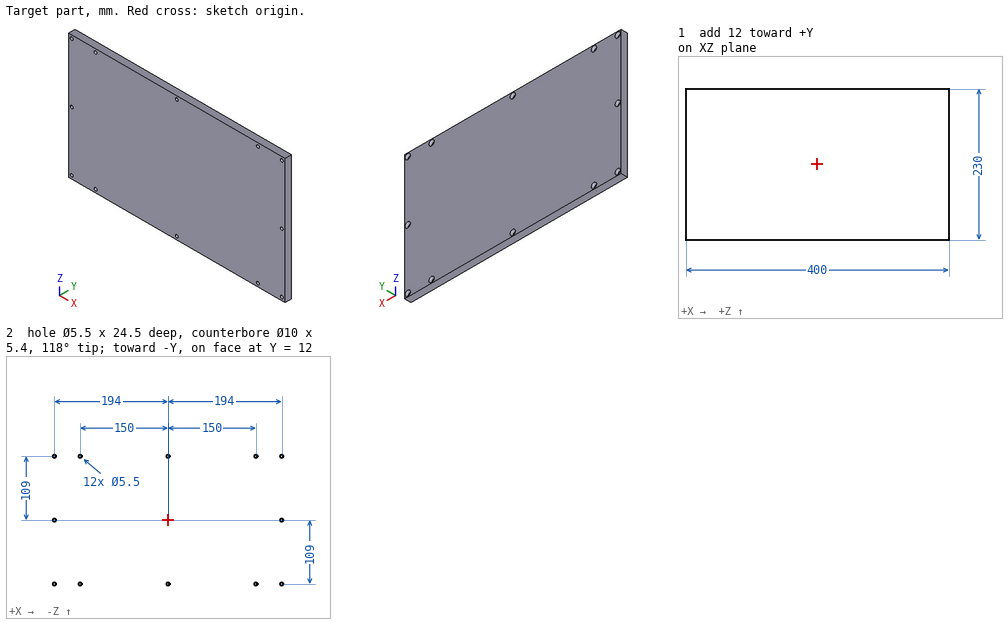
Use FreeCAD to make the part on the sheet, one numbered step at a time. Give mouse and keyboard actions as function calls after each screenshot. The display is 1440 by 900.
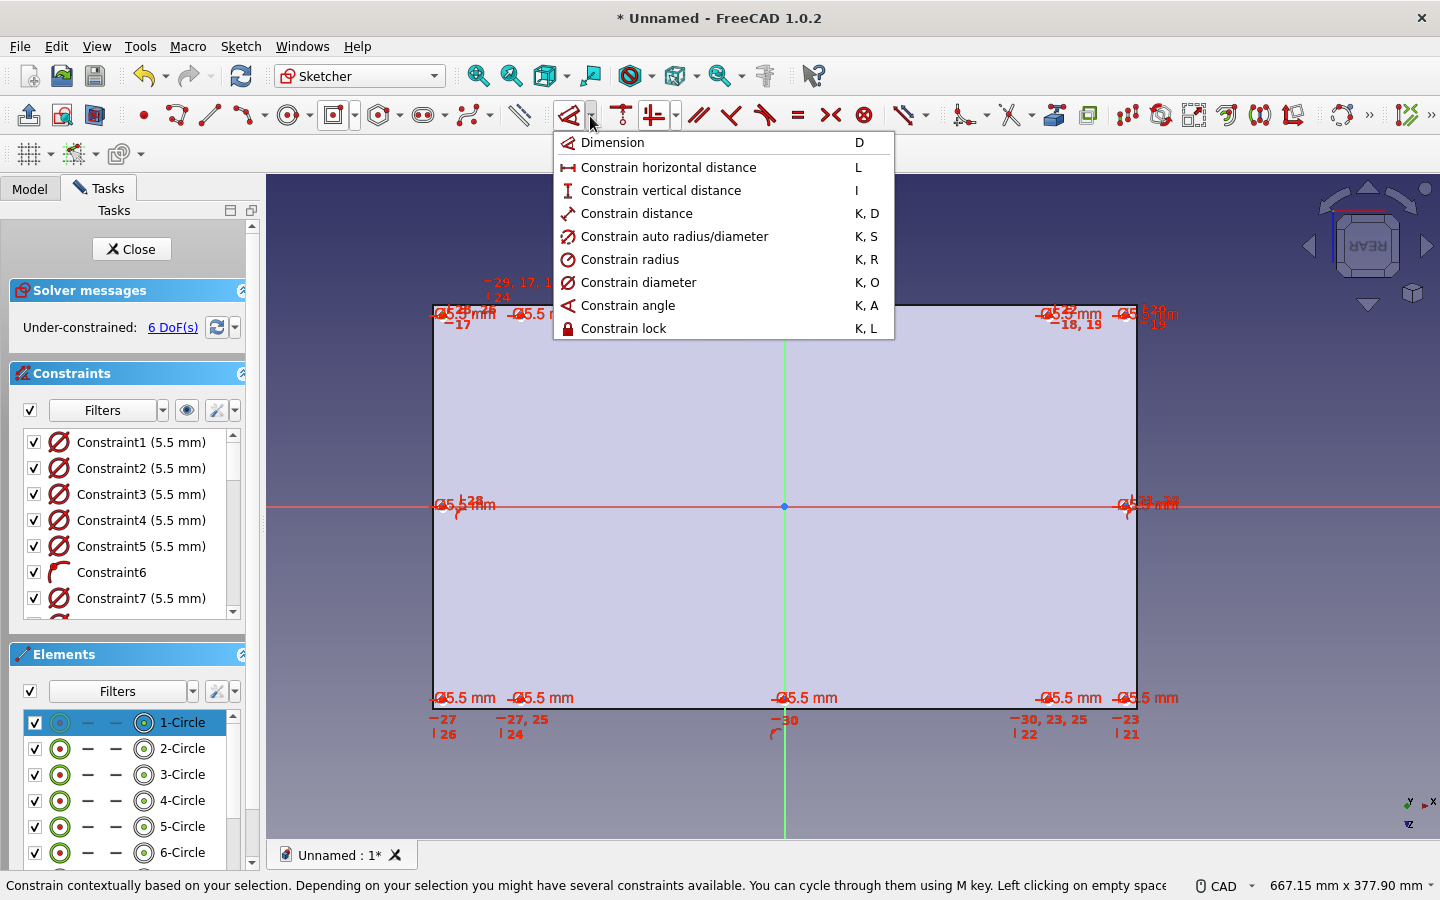
click(724, 168)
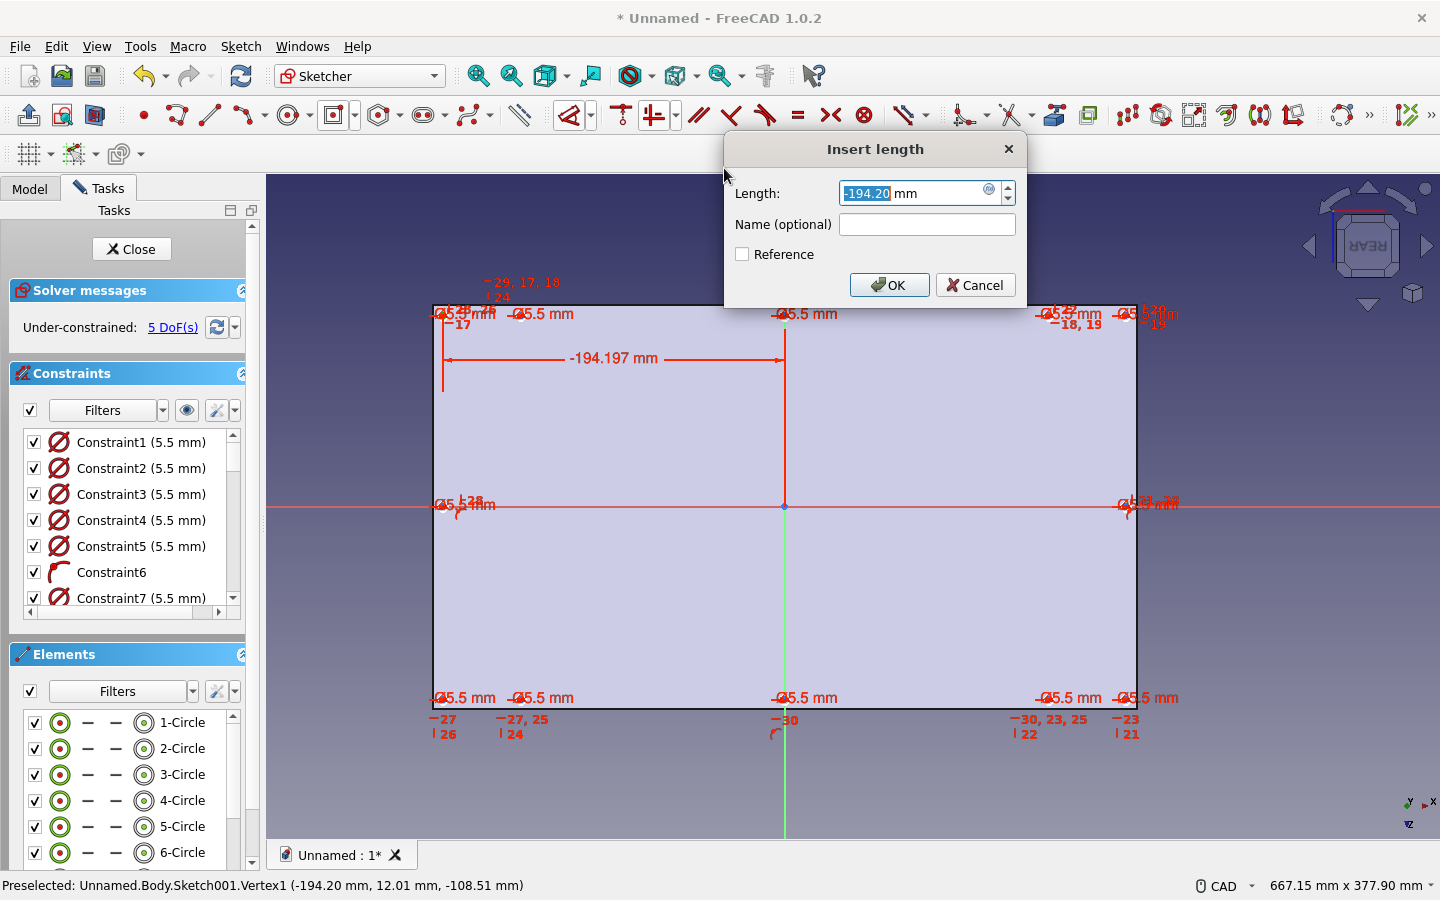
text(-194)
key(Return)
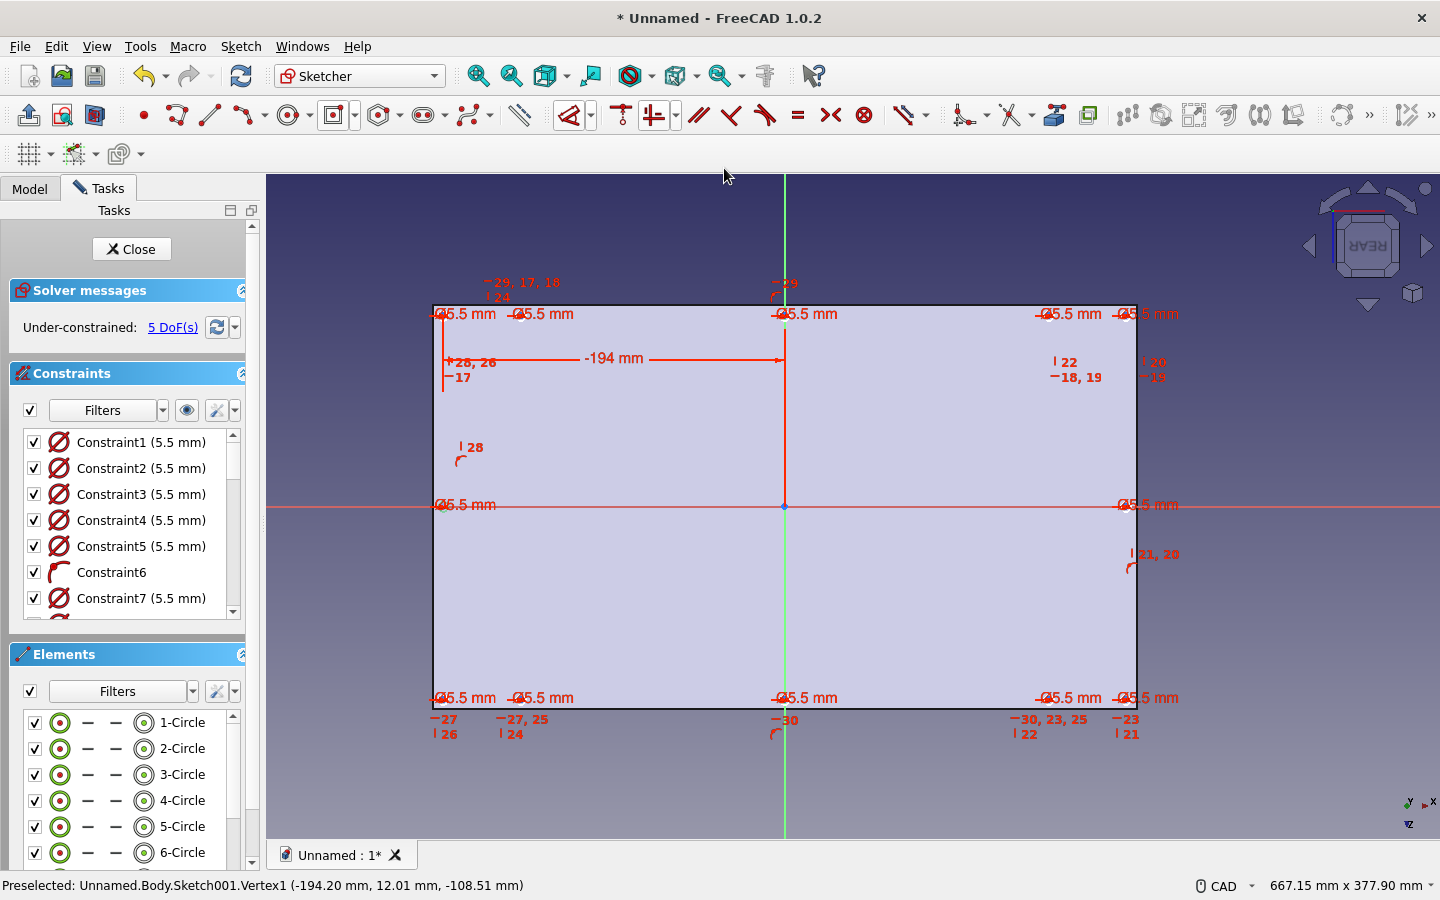
click(443, 316)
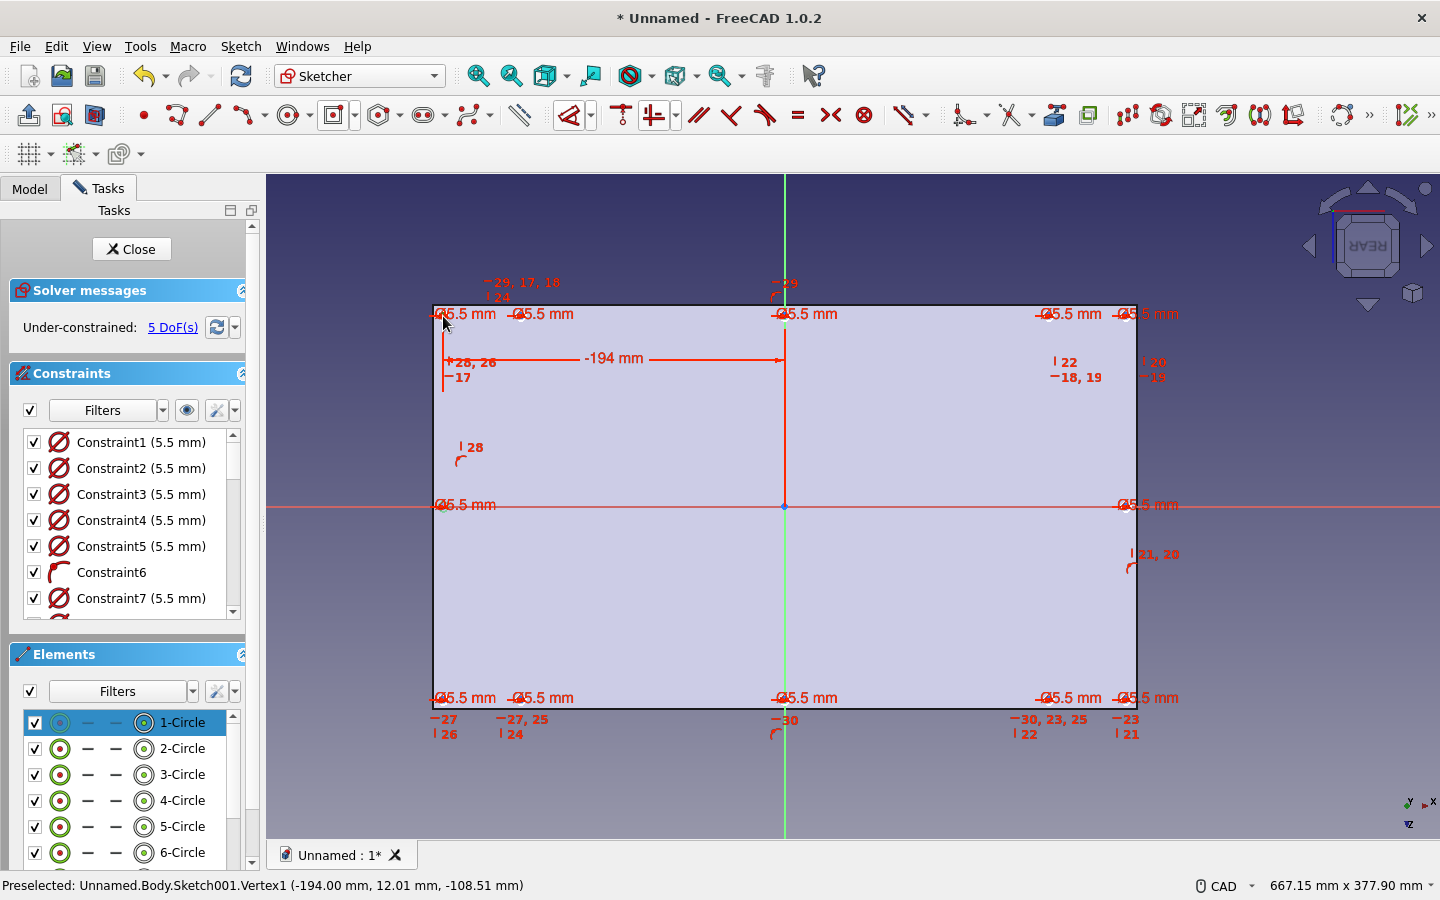
key(i)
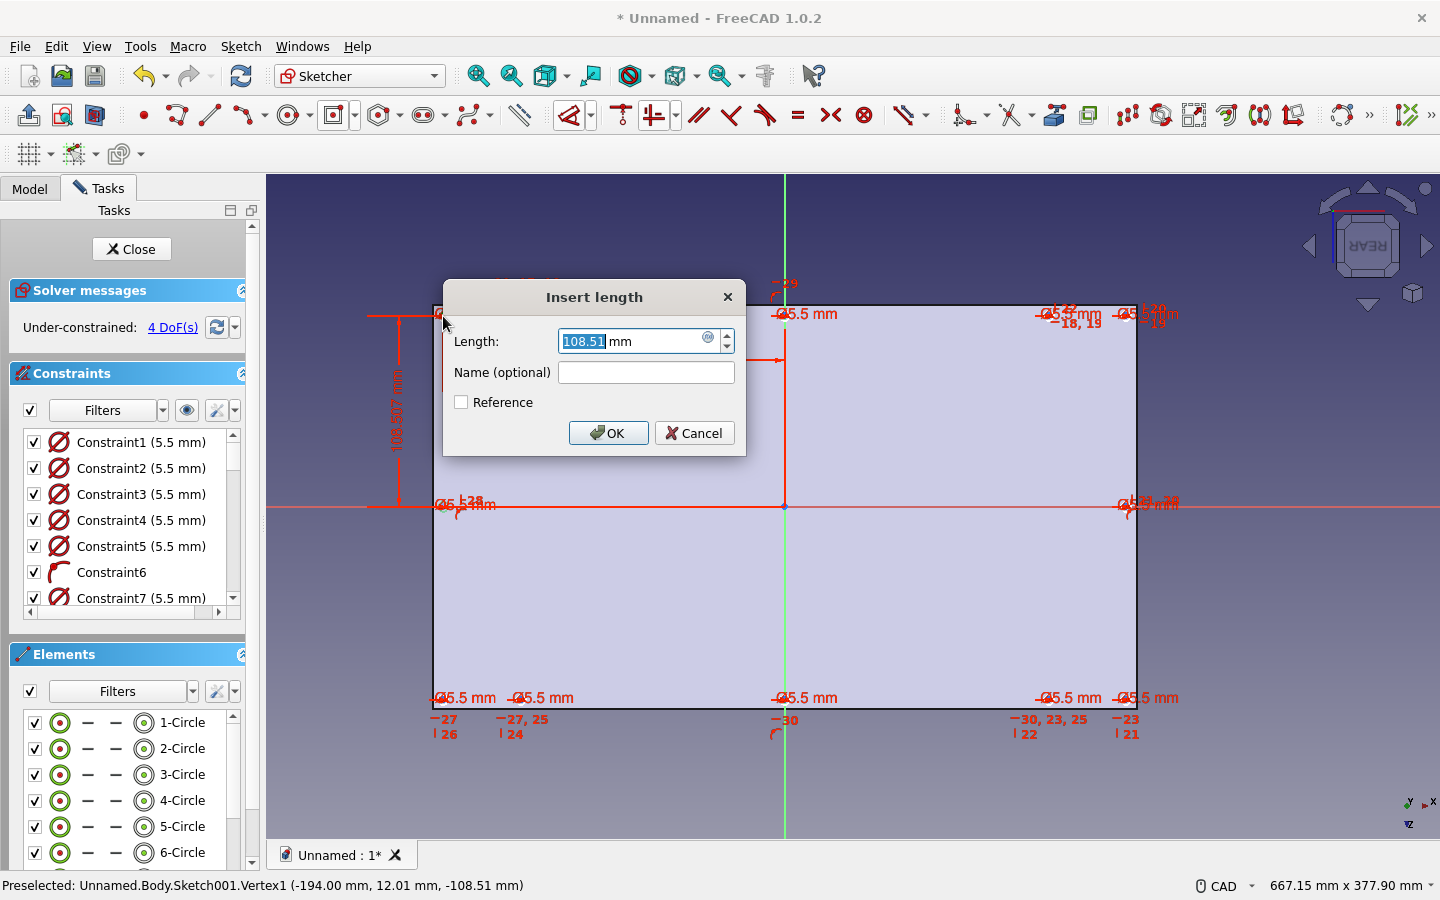
text(109)
key(Return)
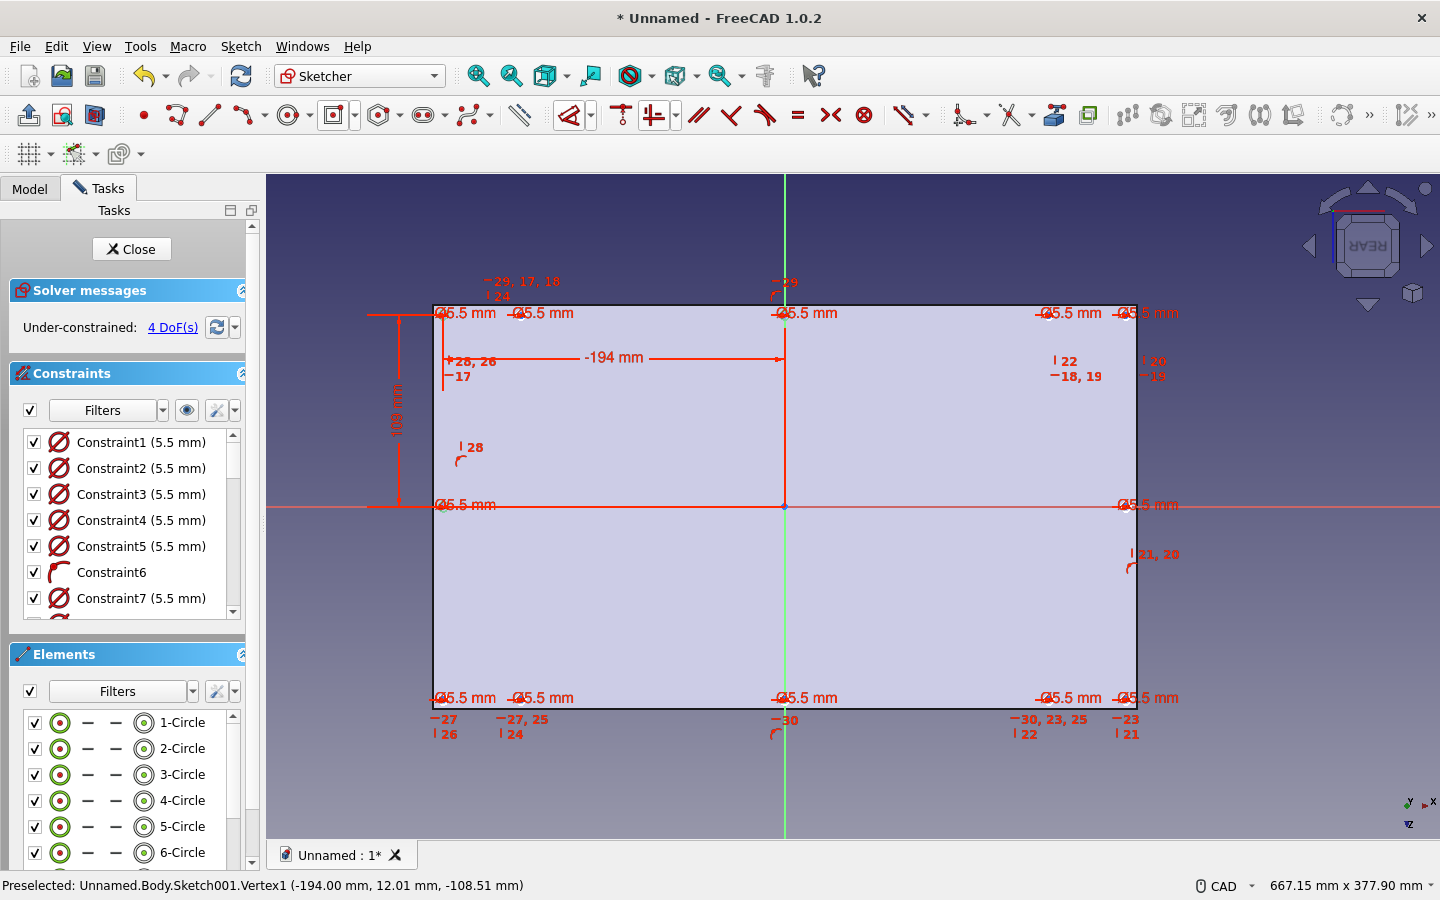
click(521, 315)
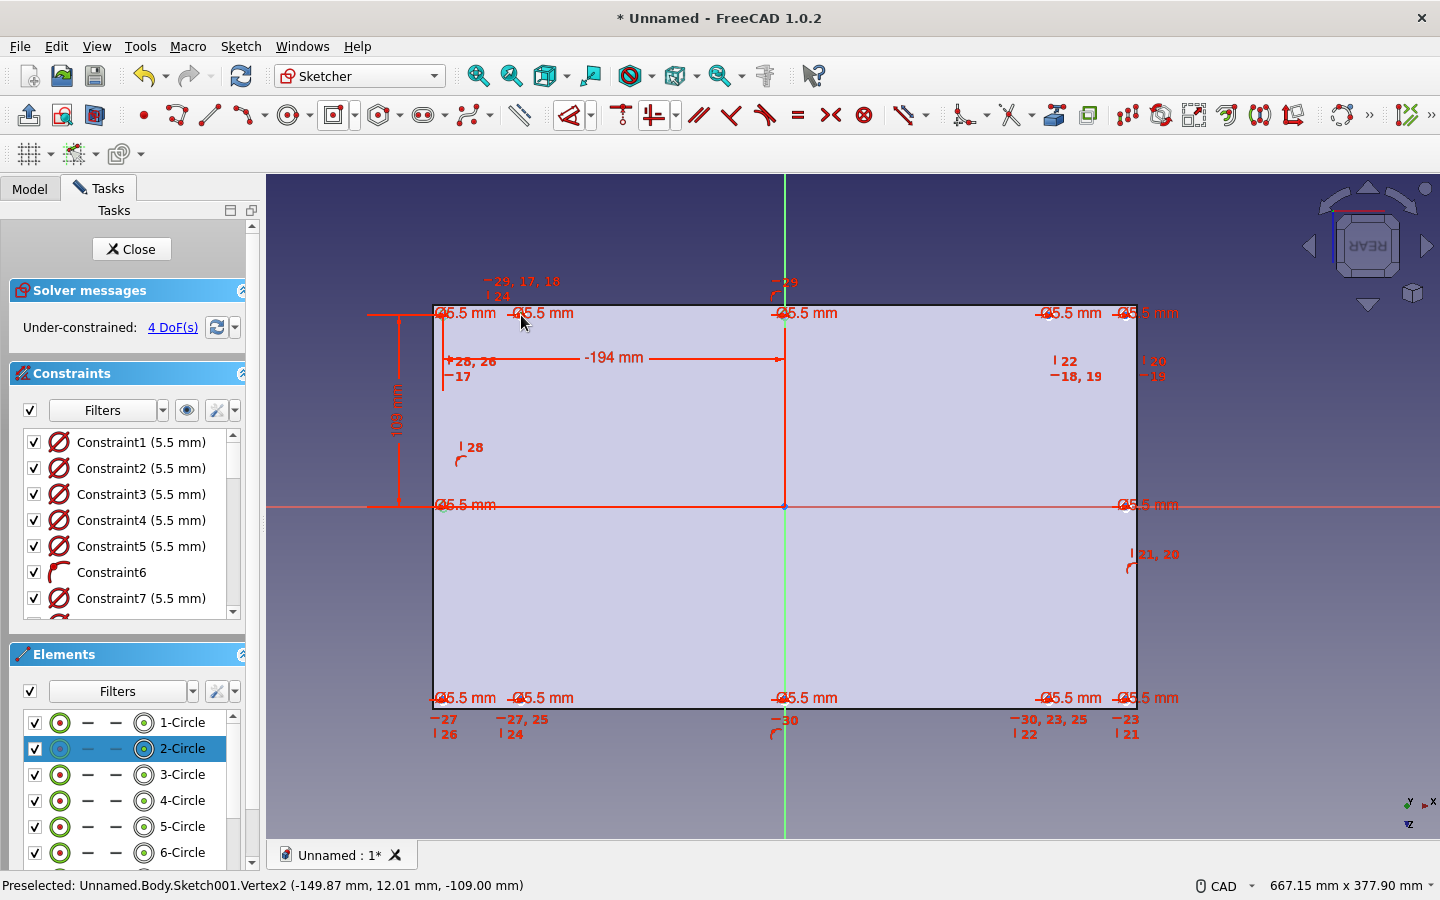
key(l)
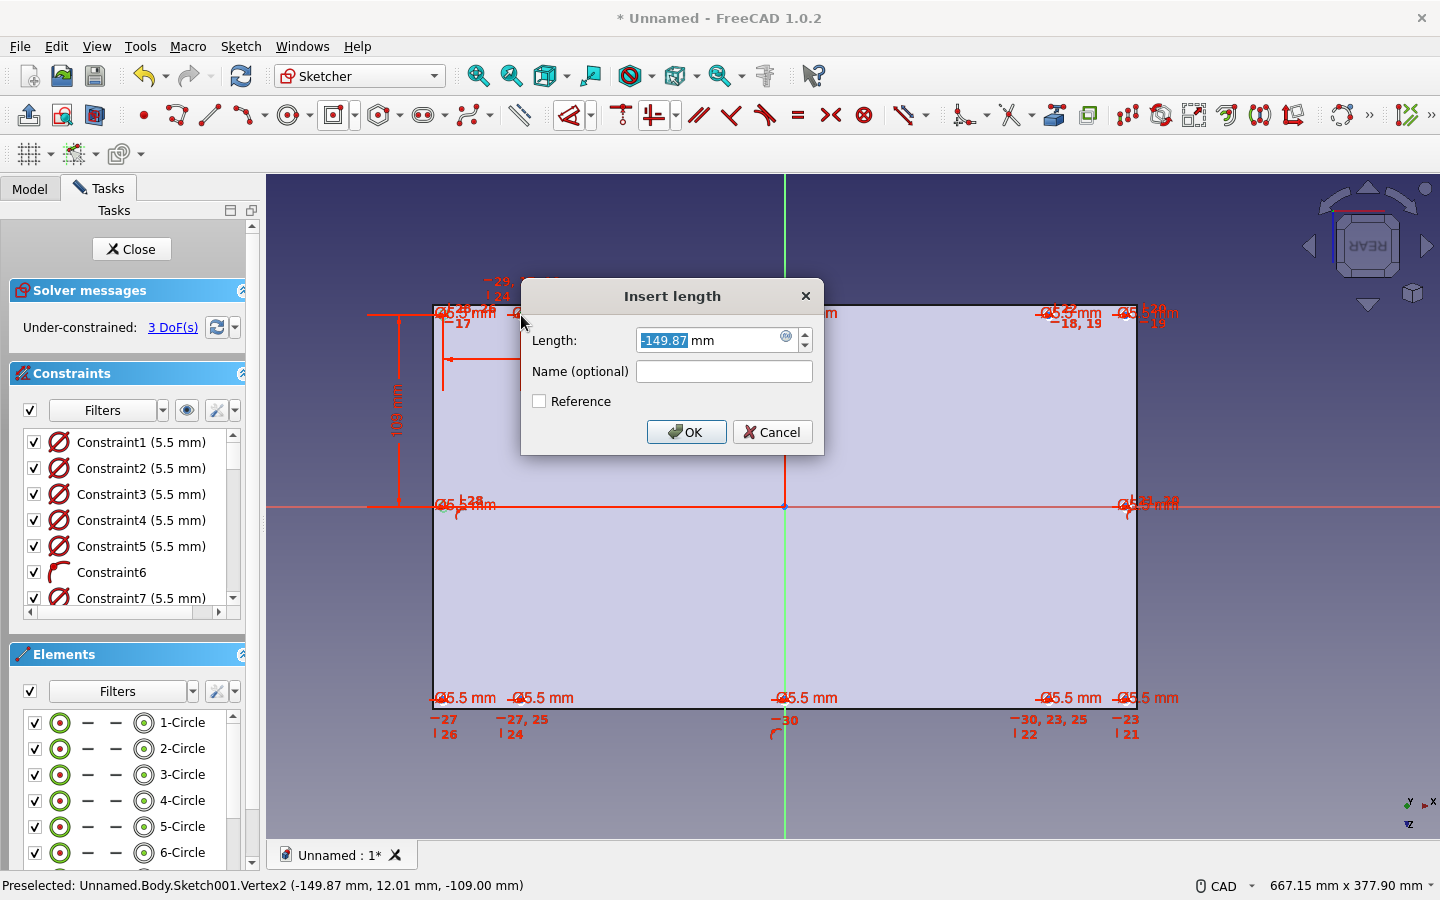
text(-150)
key(Return)